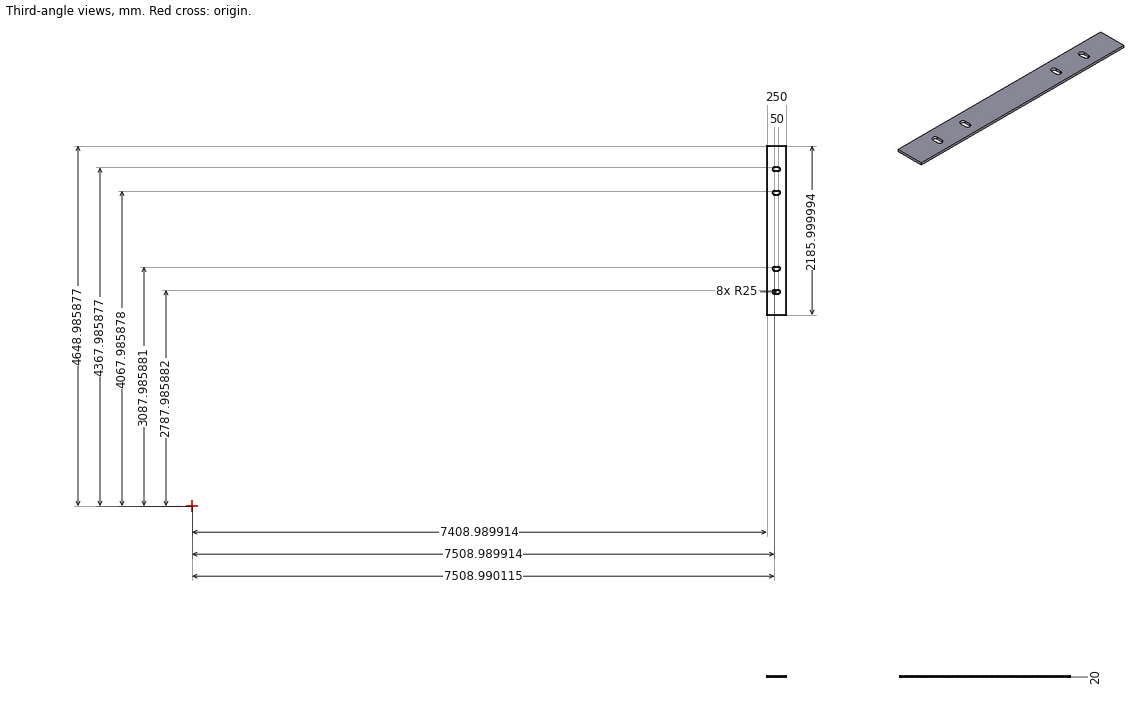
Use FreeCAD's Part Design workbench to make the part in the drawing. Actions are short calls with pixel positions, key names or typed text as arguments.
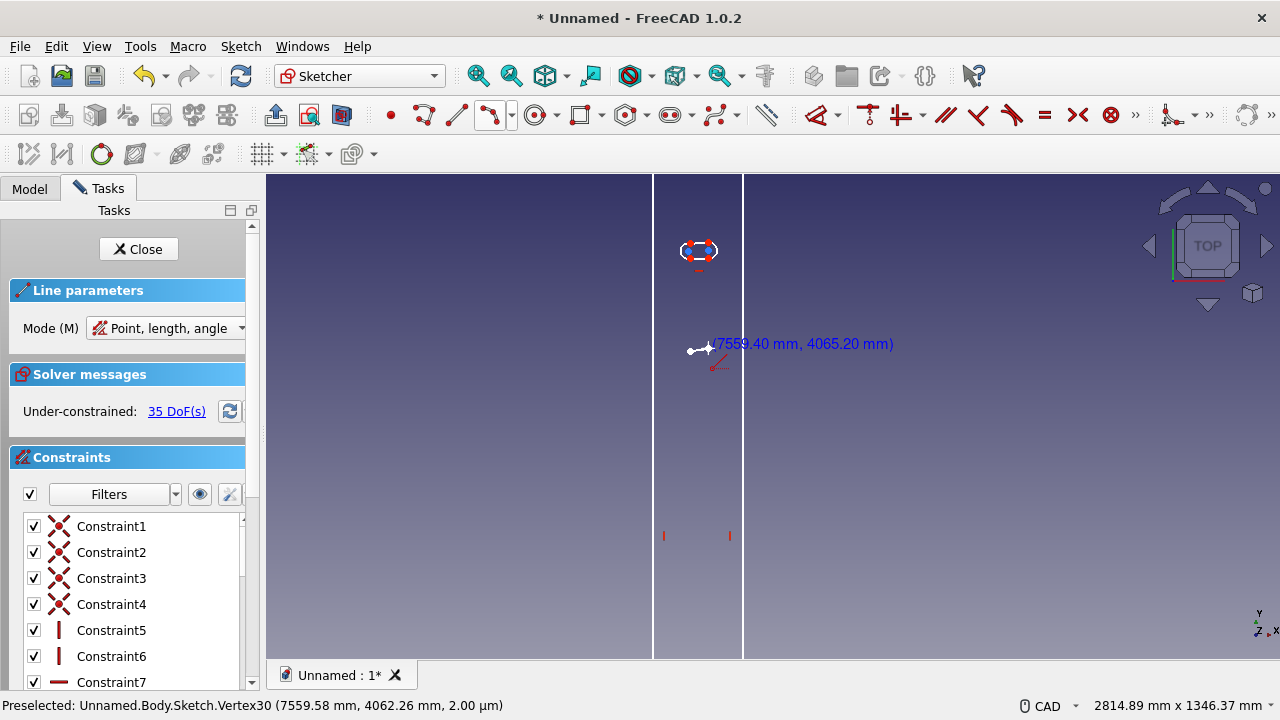
click(708, 366)
click(690, 366)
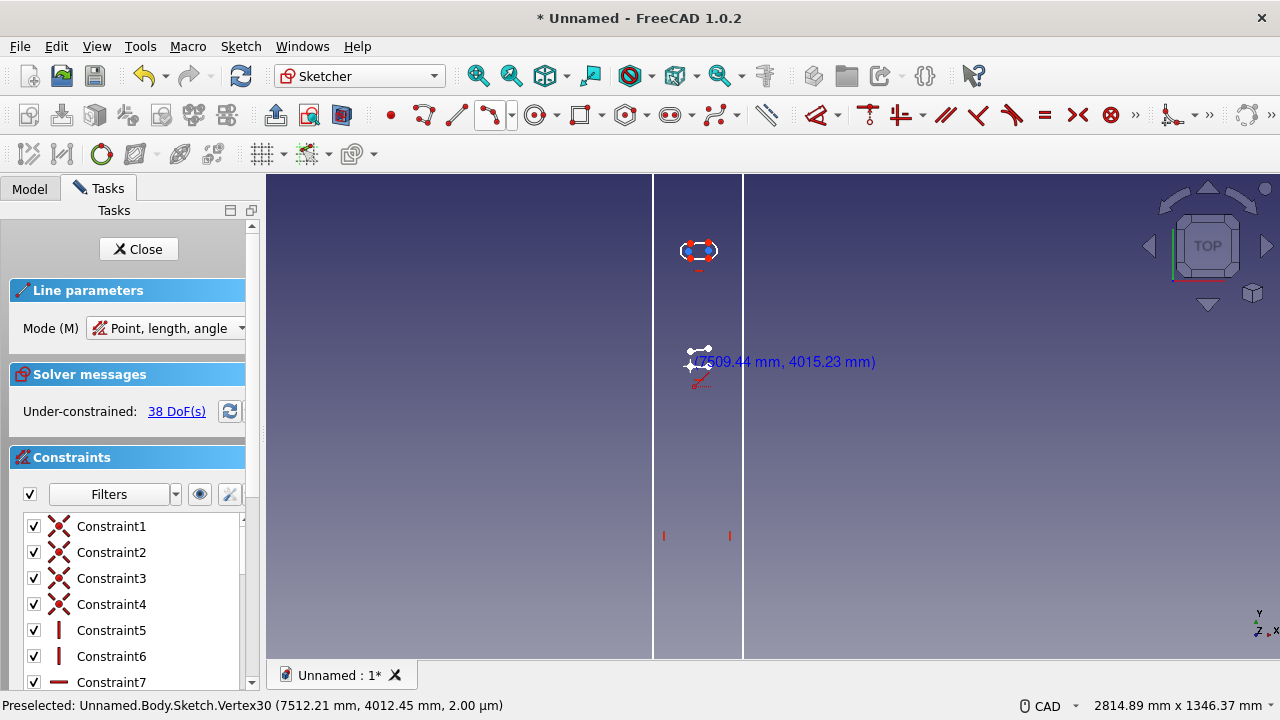
key(g)
key(3)
key(a)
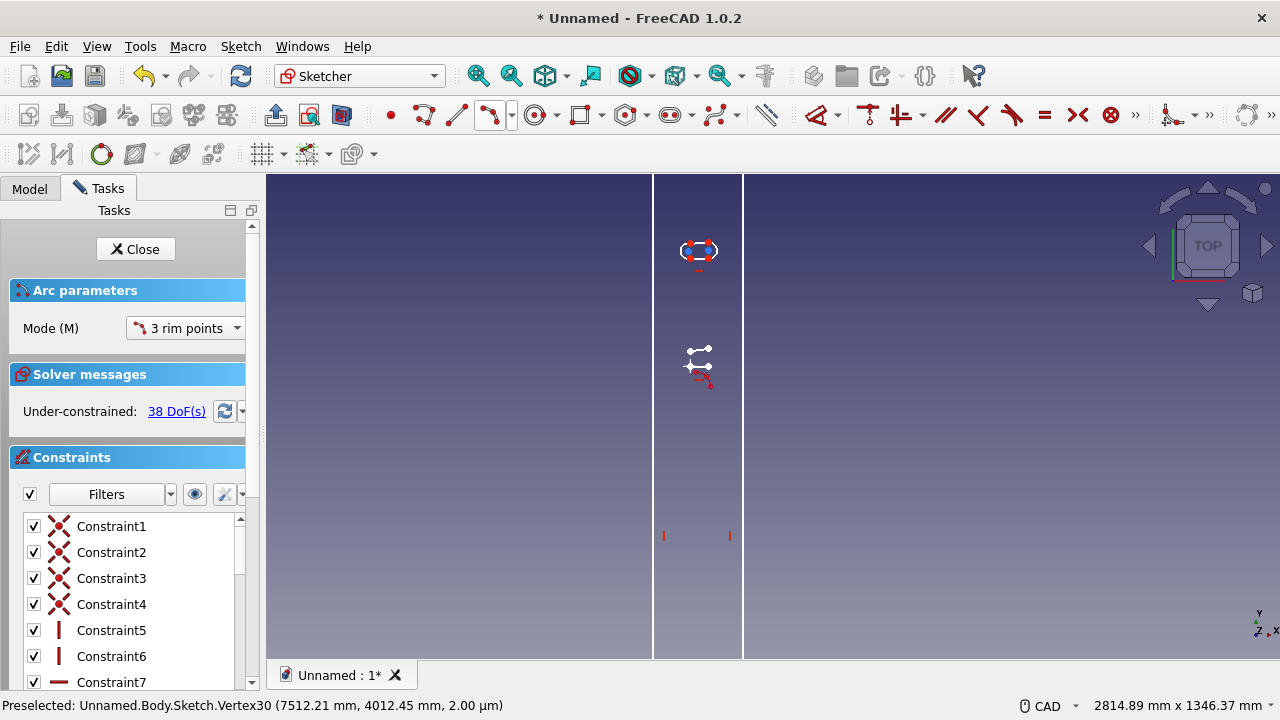
scroll(708, 348, up, 3)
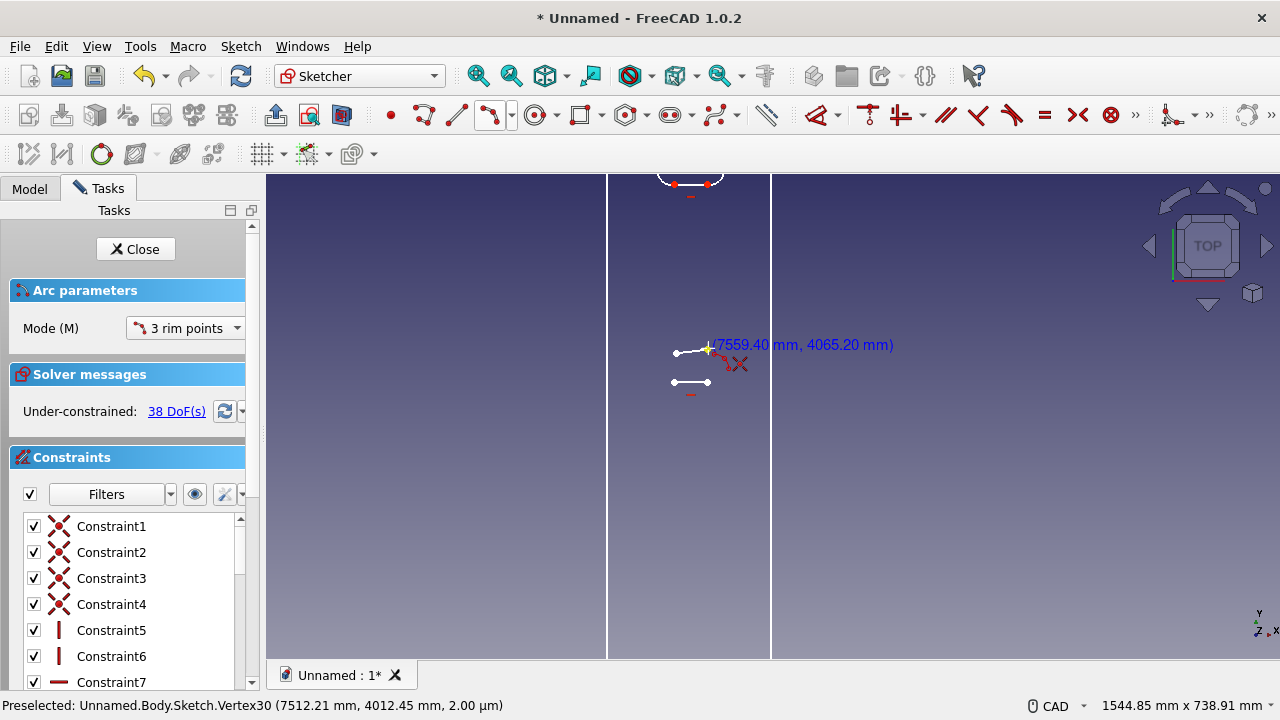
click(708, 350)
click(708, 382)
click(724, 364)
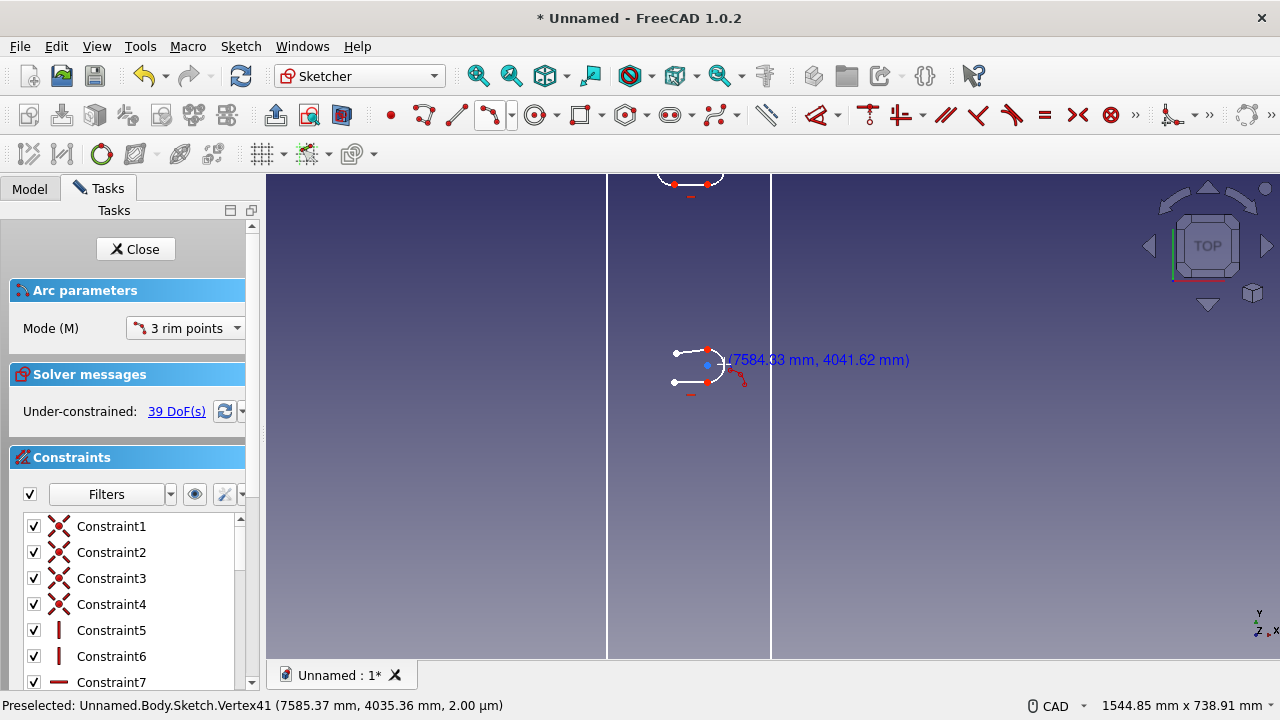
click(675, 382)
click(677, 353)
click(658, 364)
key(Escape)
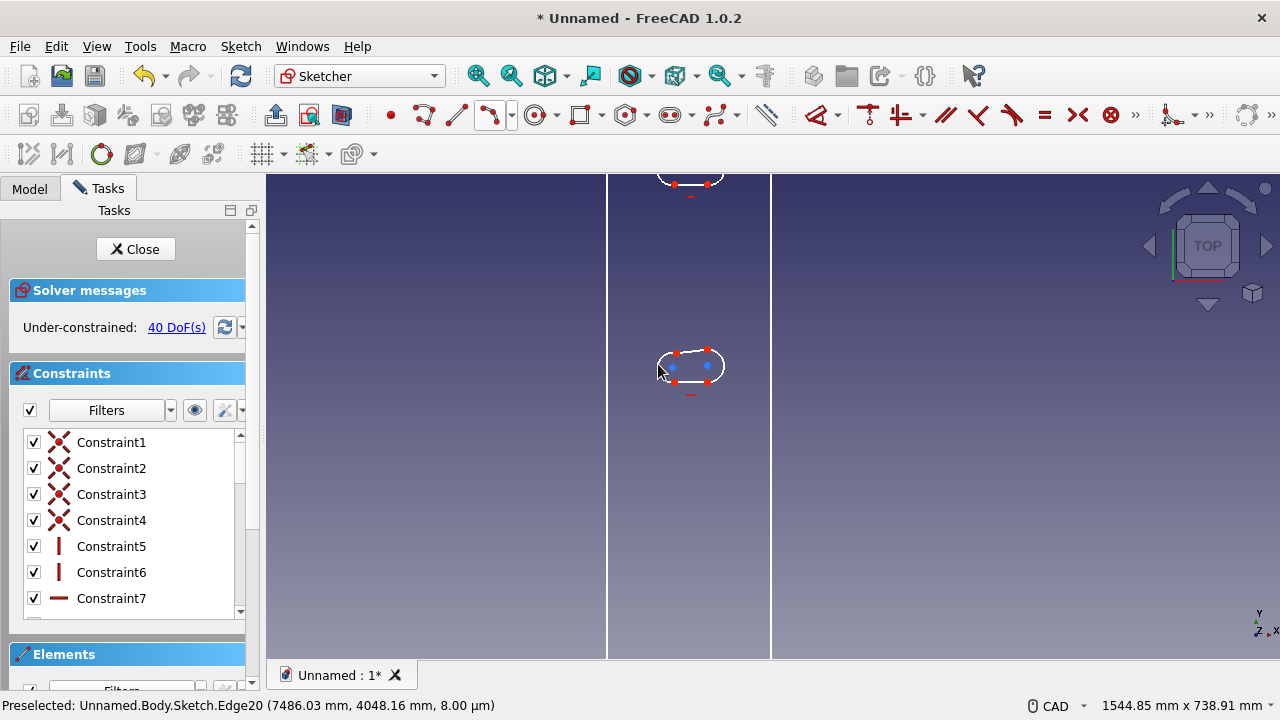
scroll(708, 349, down, 8)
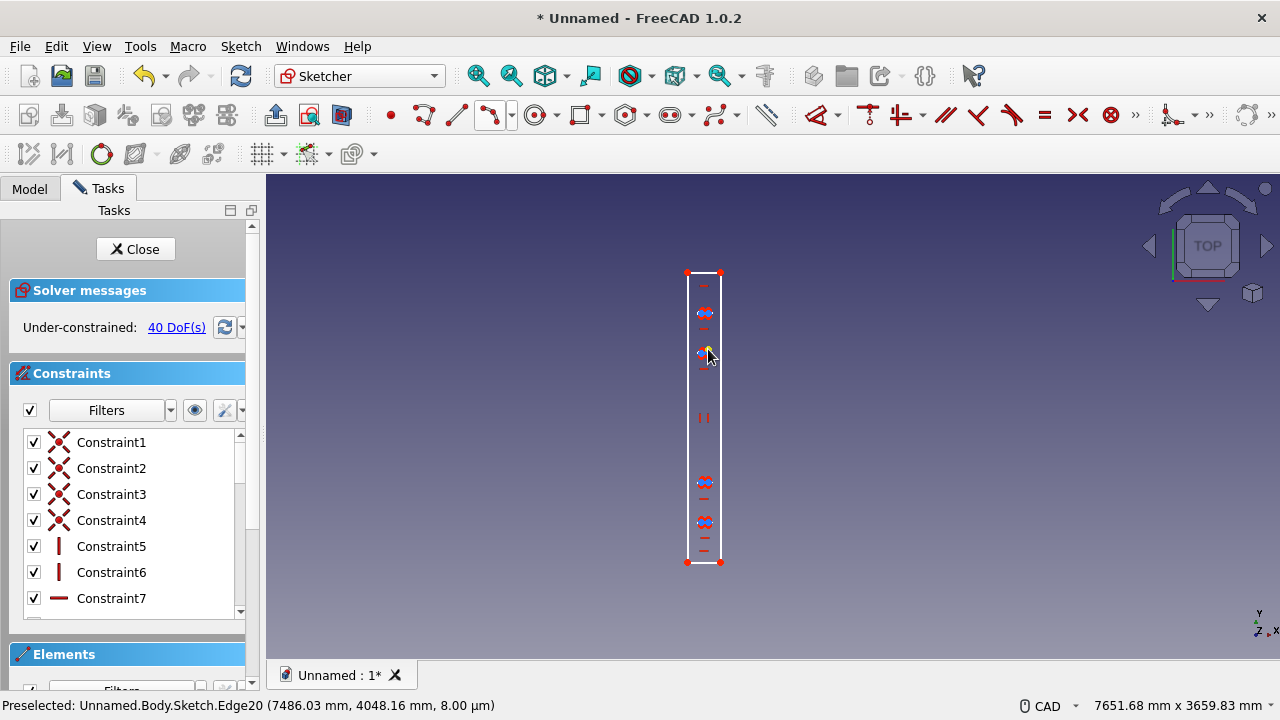
scroll(704, 520, up, 10)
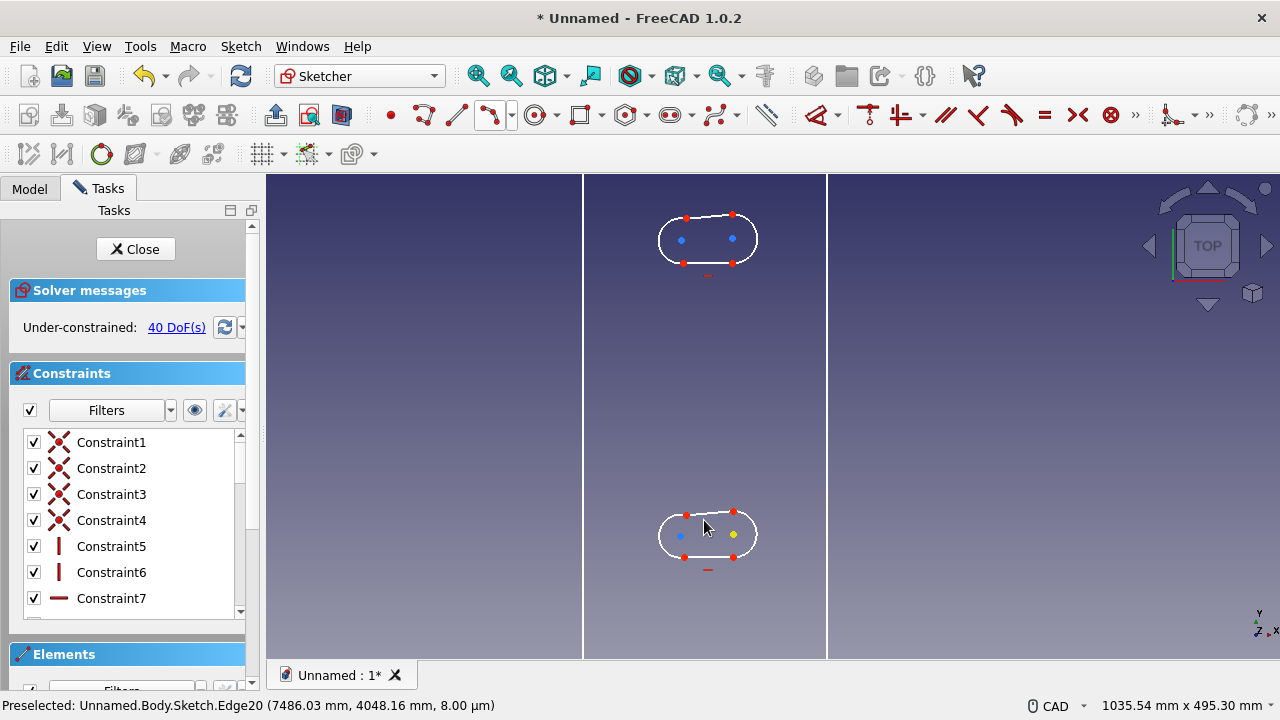
click(701, 514)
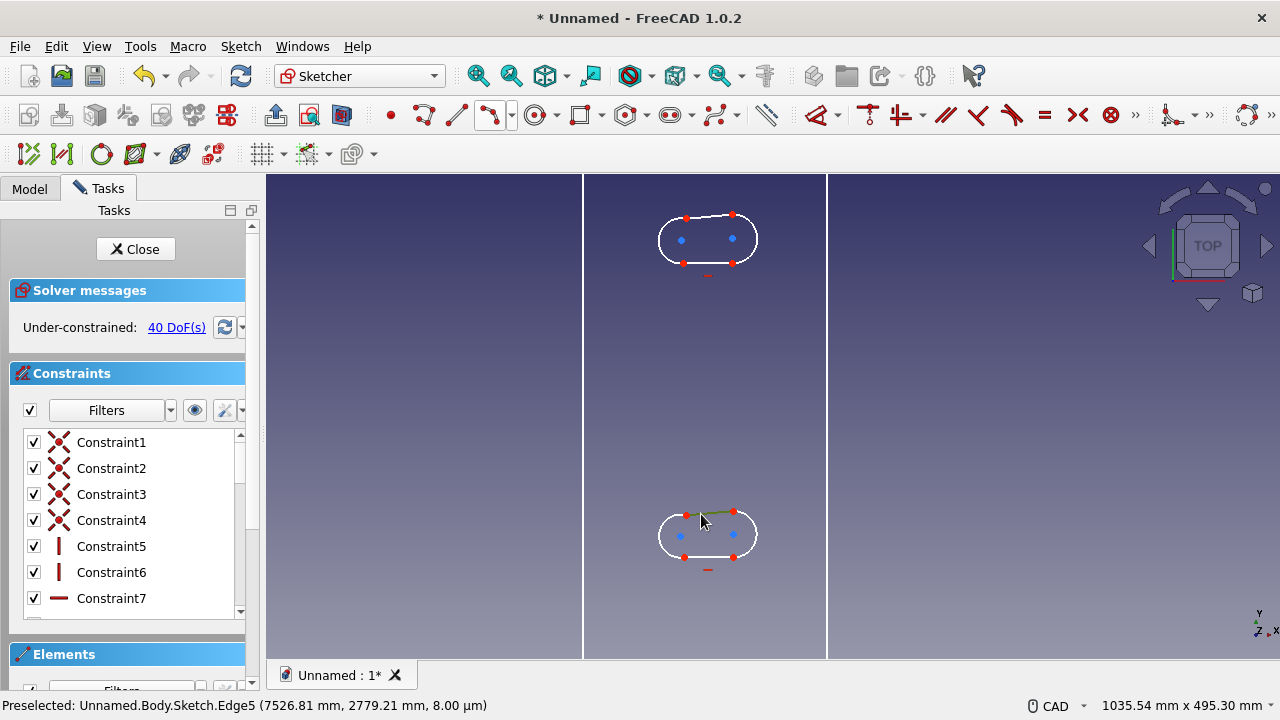
click(752, 548)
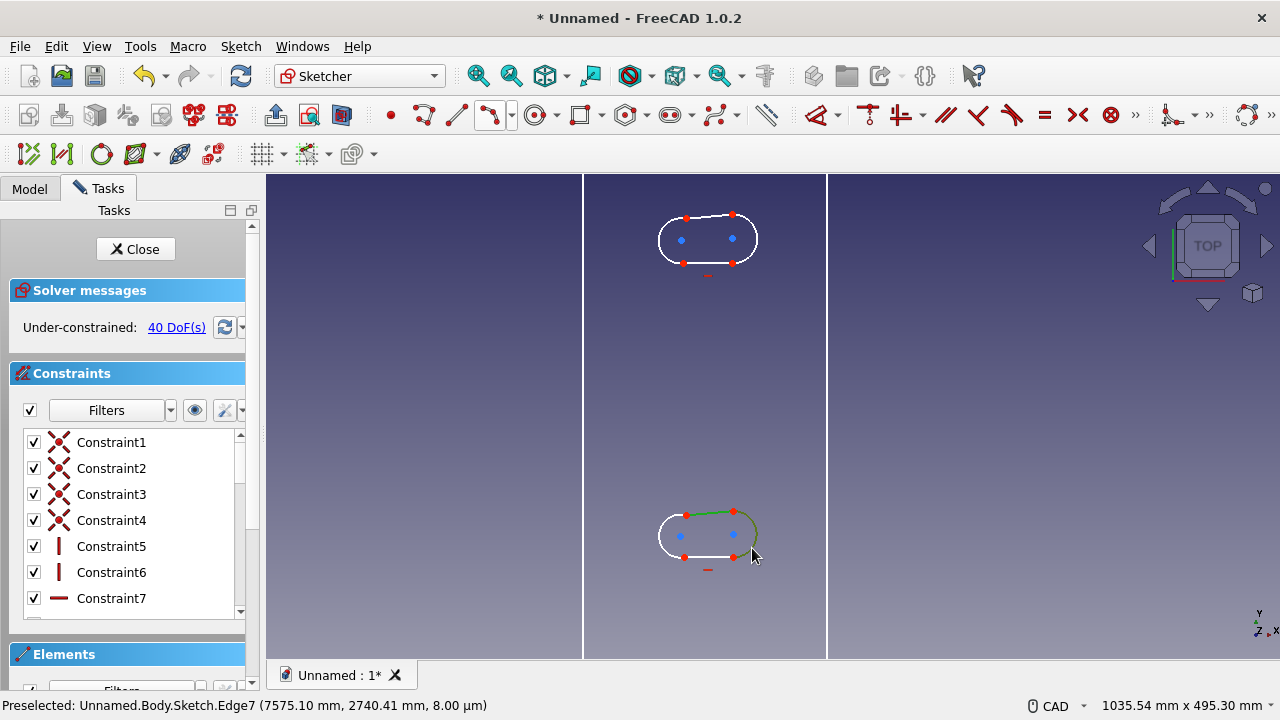
key(t)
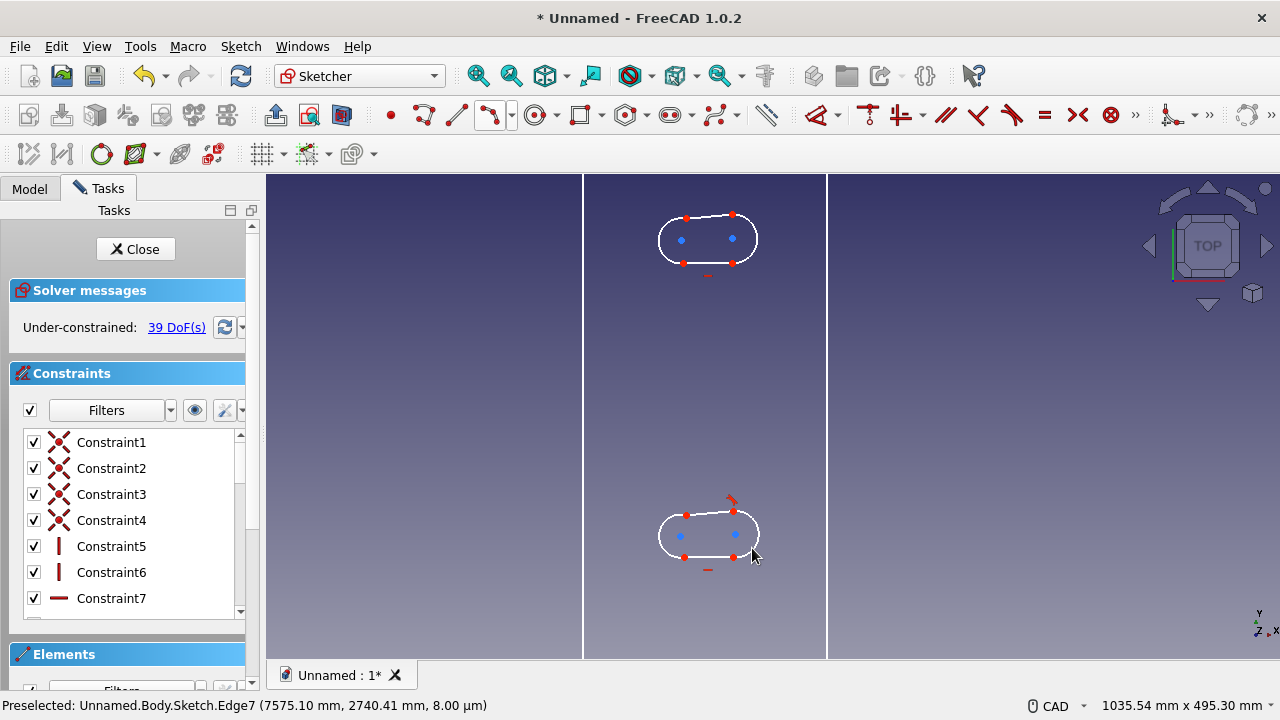
click(701, 514)